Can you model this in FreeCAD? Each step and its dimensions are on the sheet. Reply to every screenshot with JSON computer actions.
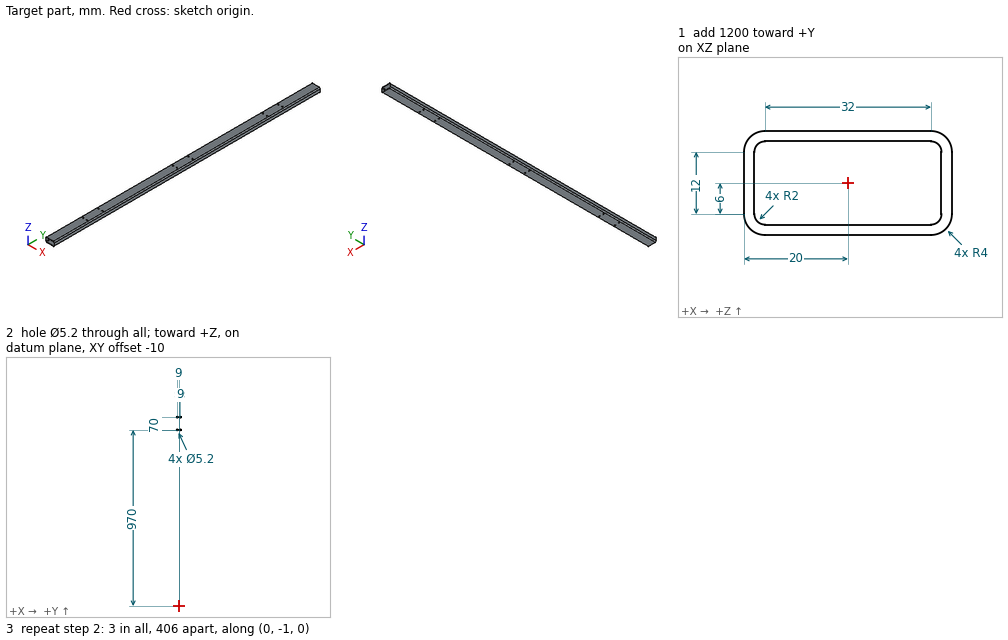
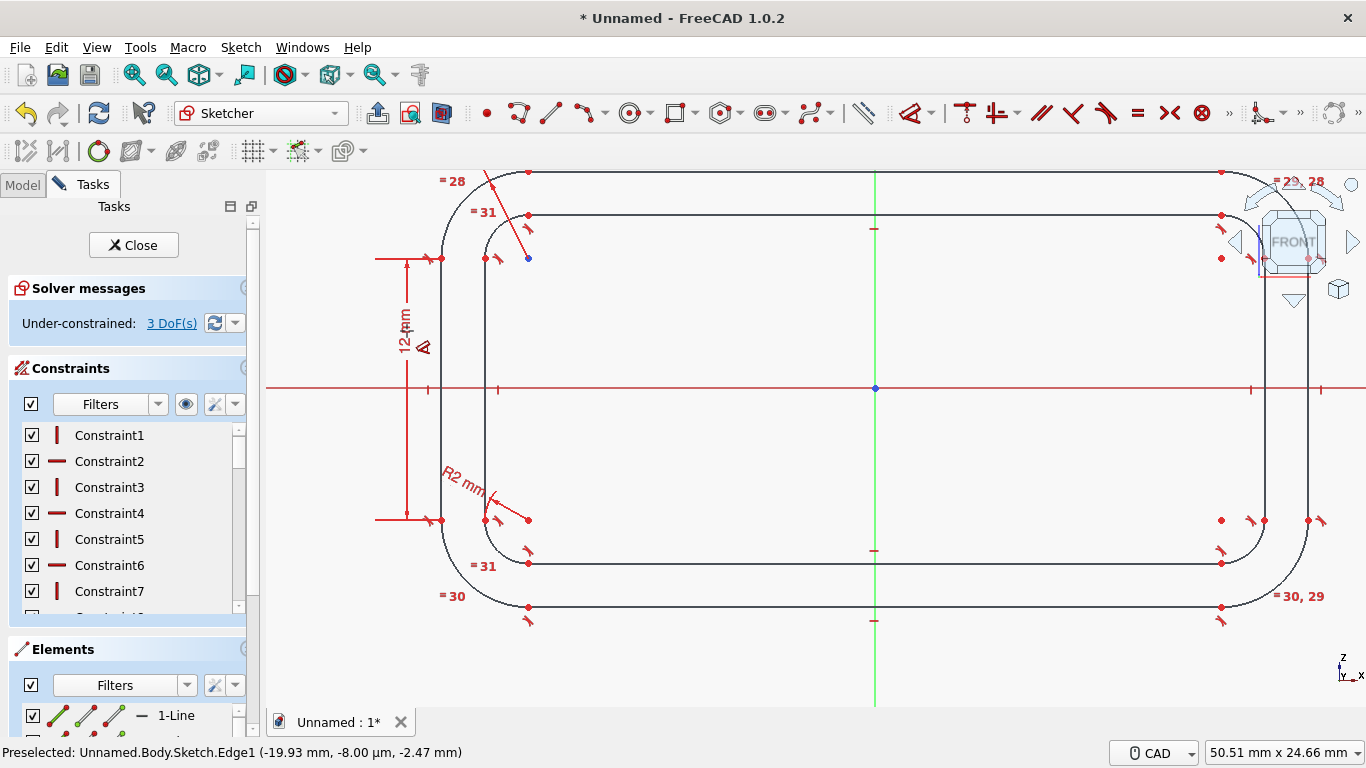
{"action": "scroll", "coordinate": [487, 541], "scroll_direction": "down", "scroll_amount": 2}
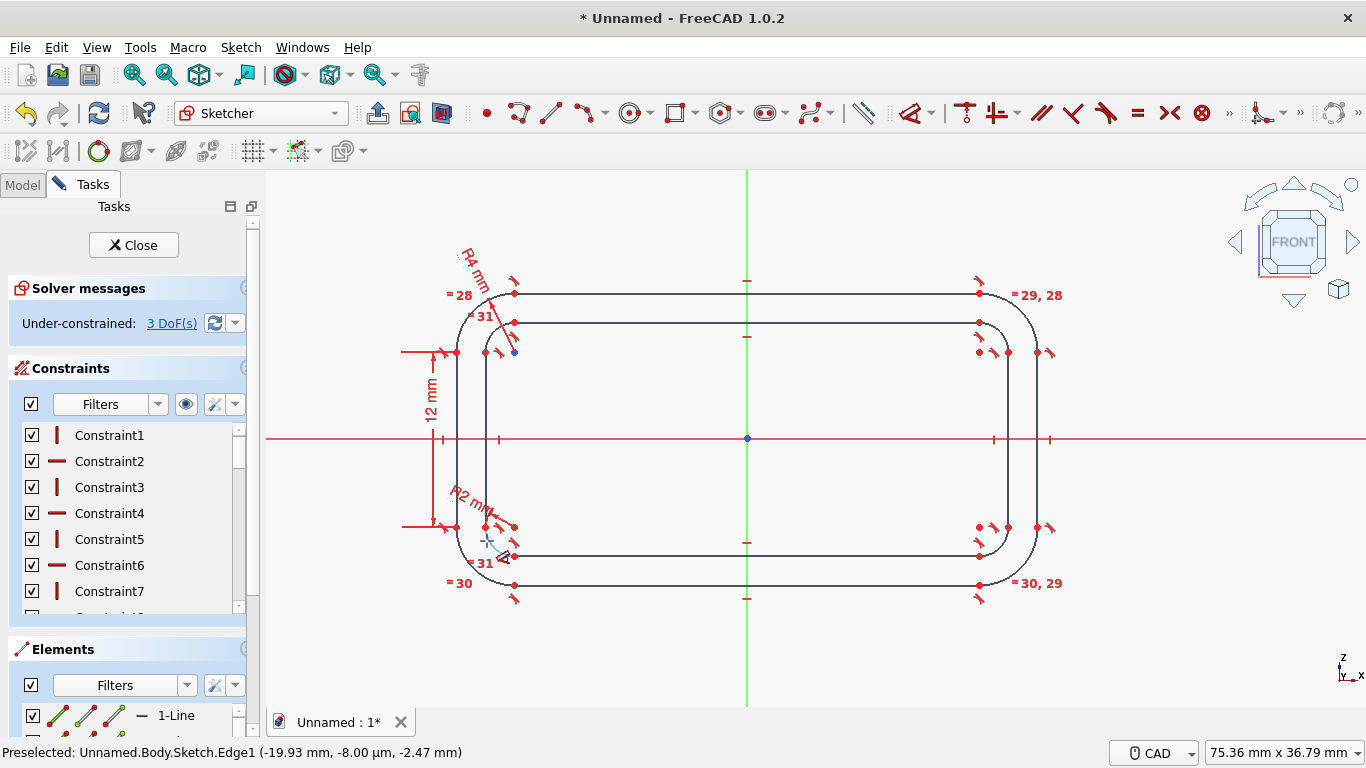
{"action": "left_click", "coordinate": [654, 294]}
{"action": "left_click", "coordinate": [640, 260]}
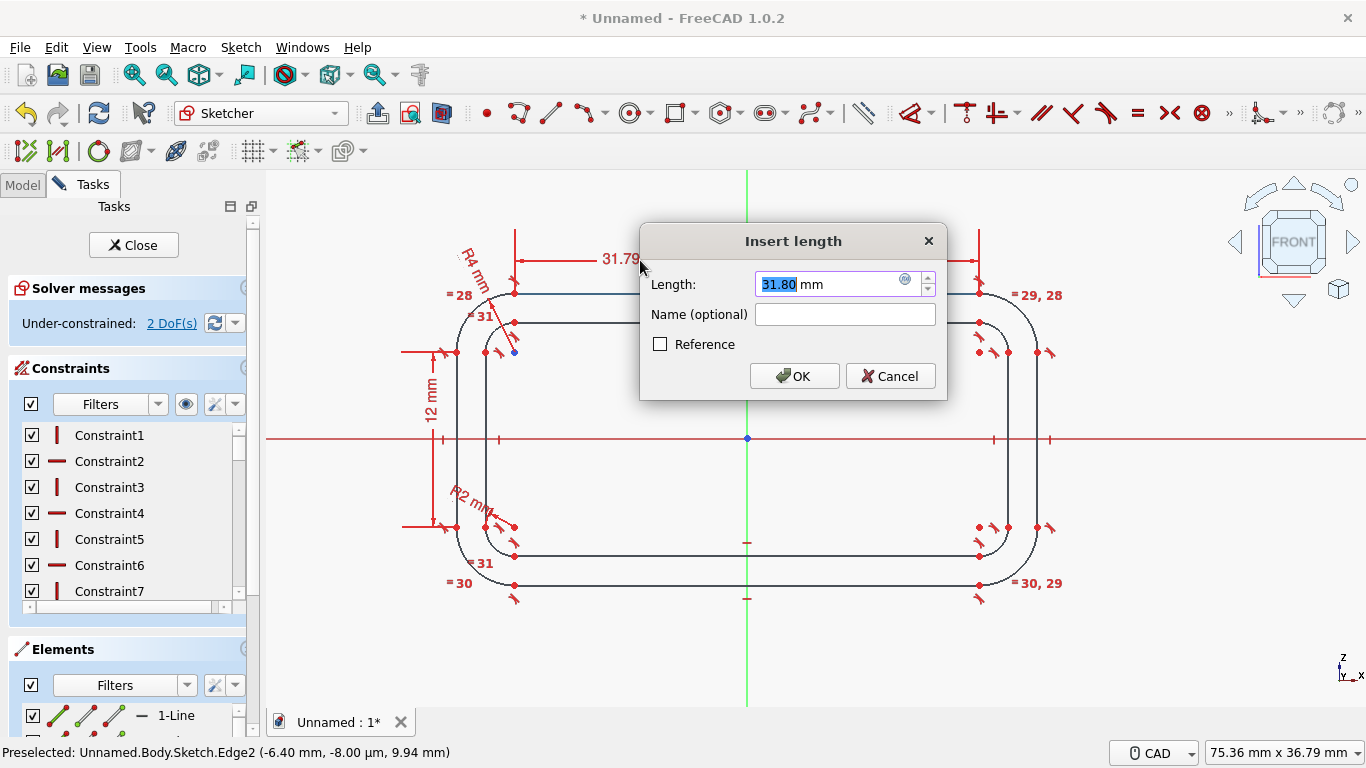
{"action": "type", "text": "32"}
{"action": "key", "text": "Return"}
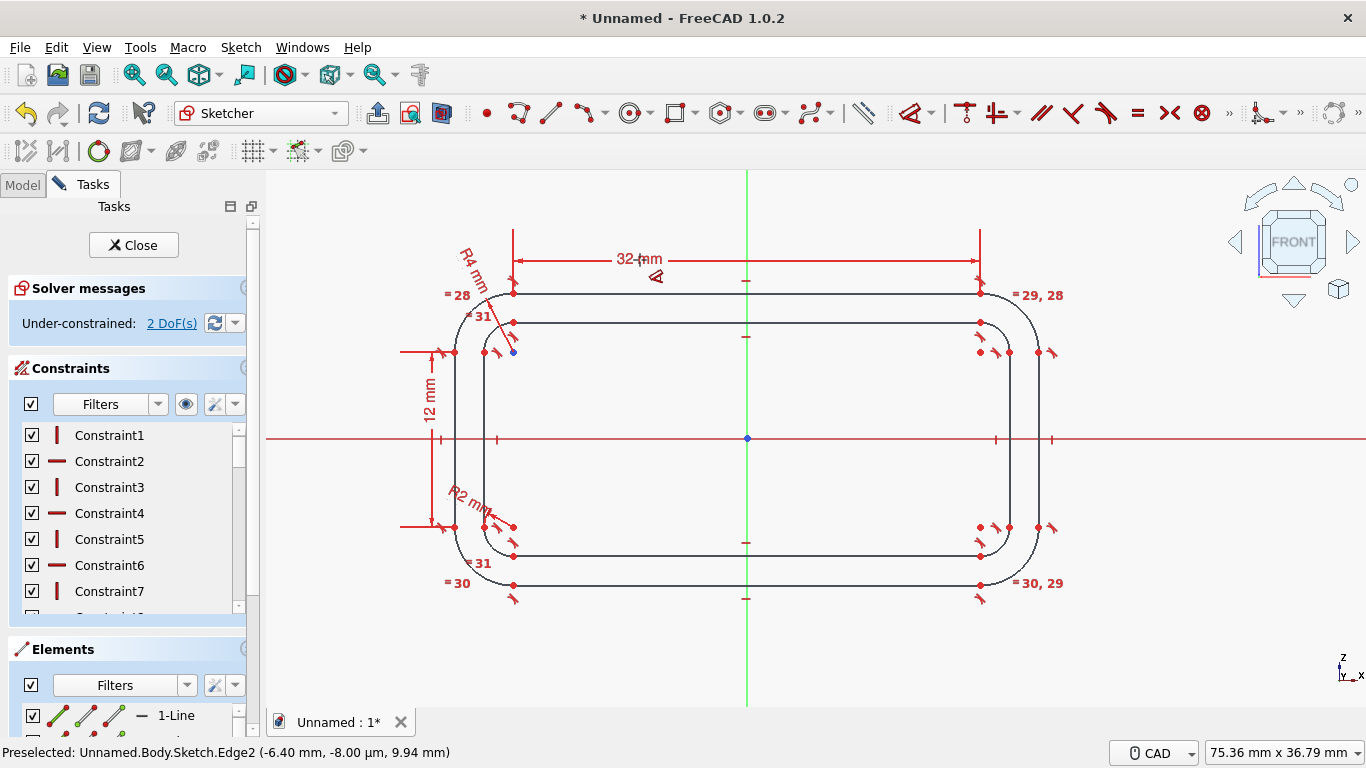
{"action": "left_click", "coordinate": [455, 527]}
{"action": "left_click", "coordinate": [421, 463]}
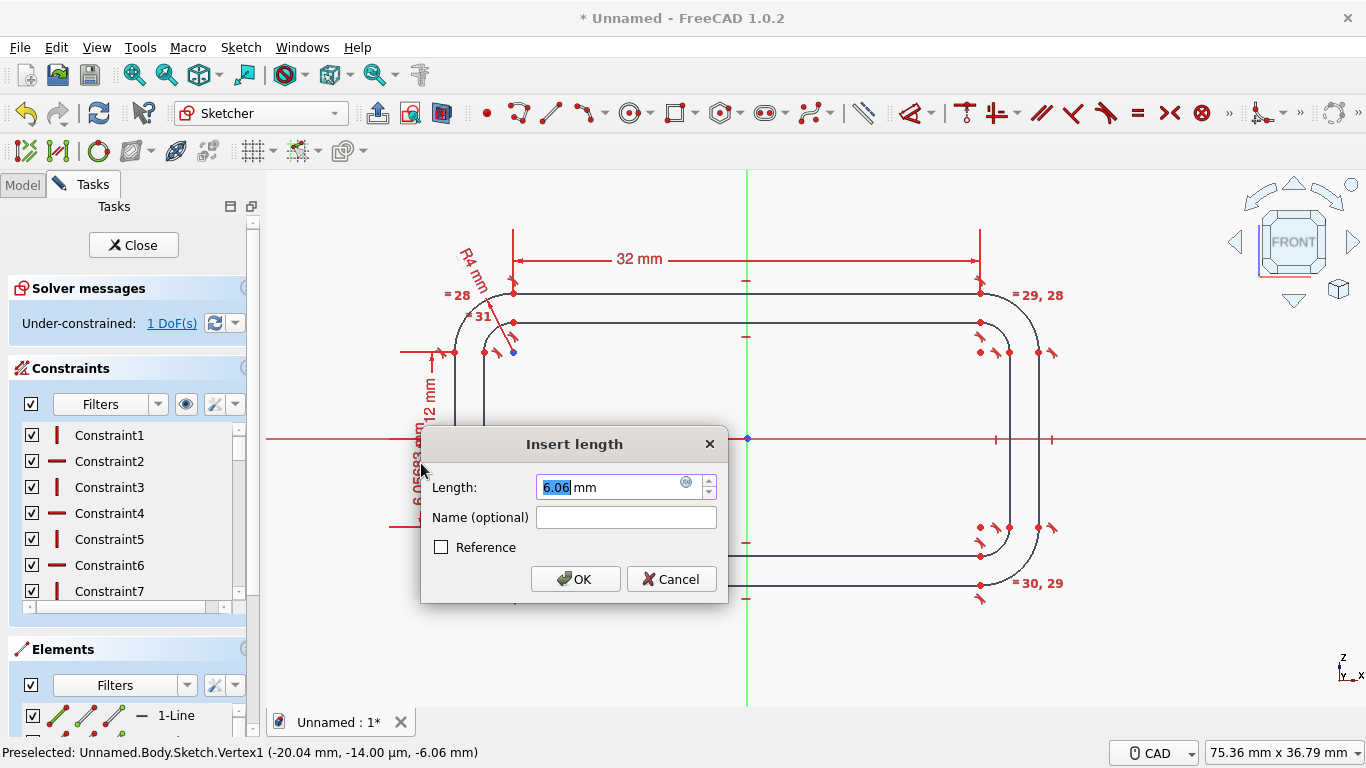
{"action": "type", "text": "6"}
{"action": "key", "text": "Return"}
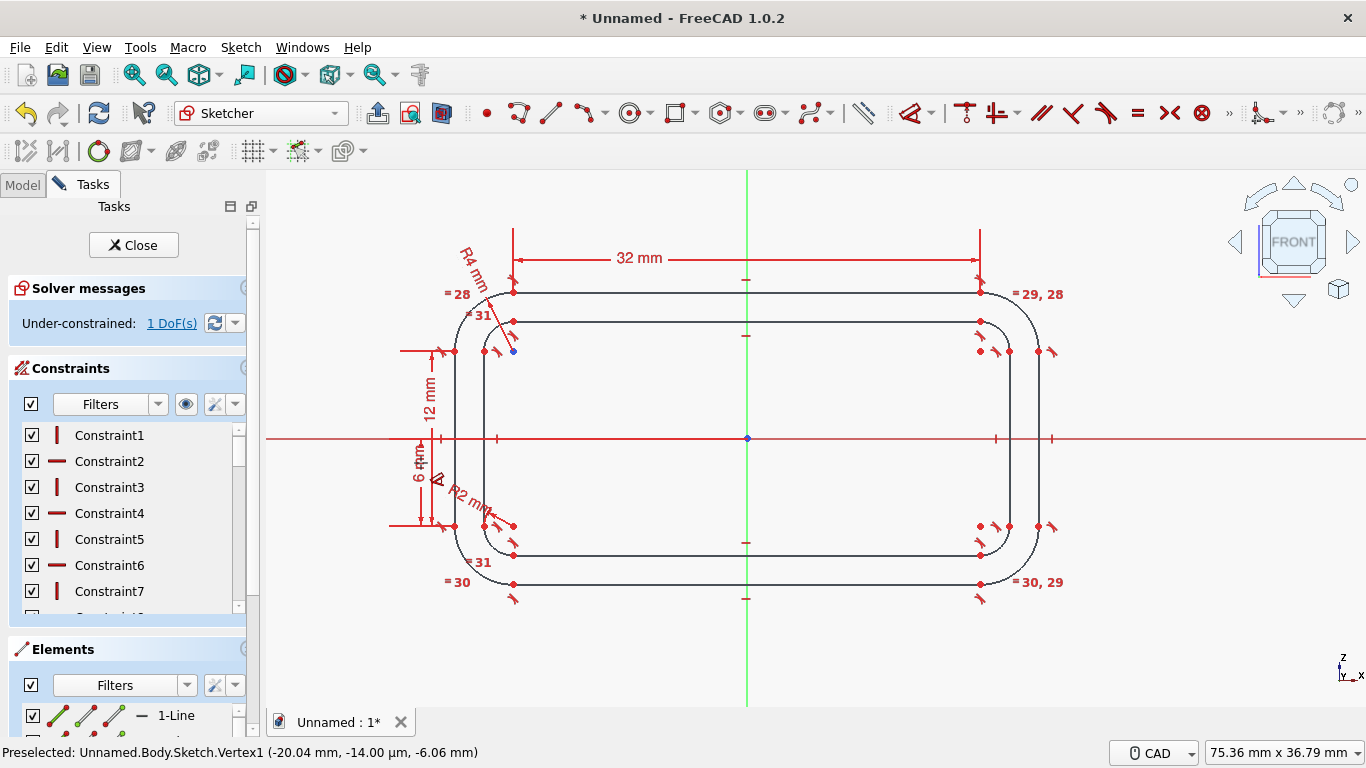
{"action": "left_click", "coordinate": [455, 526]}
{"action": "left_click", "coordinate": [601, 405]}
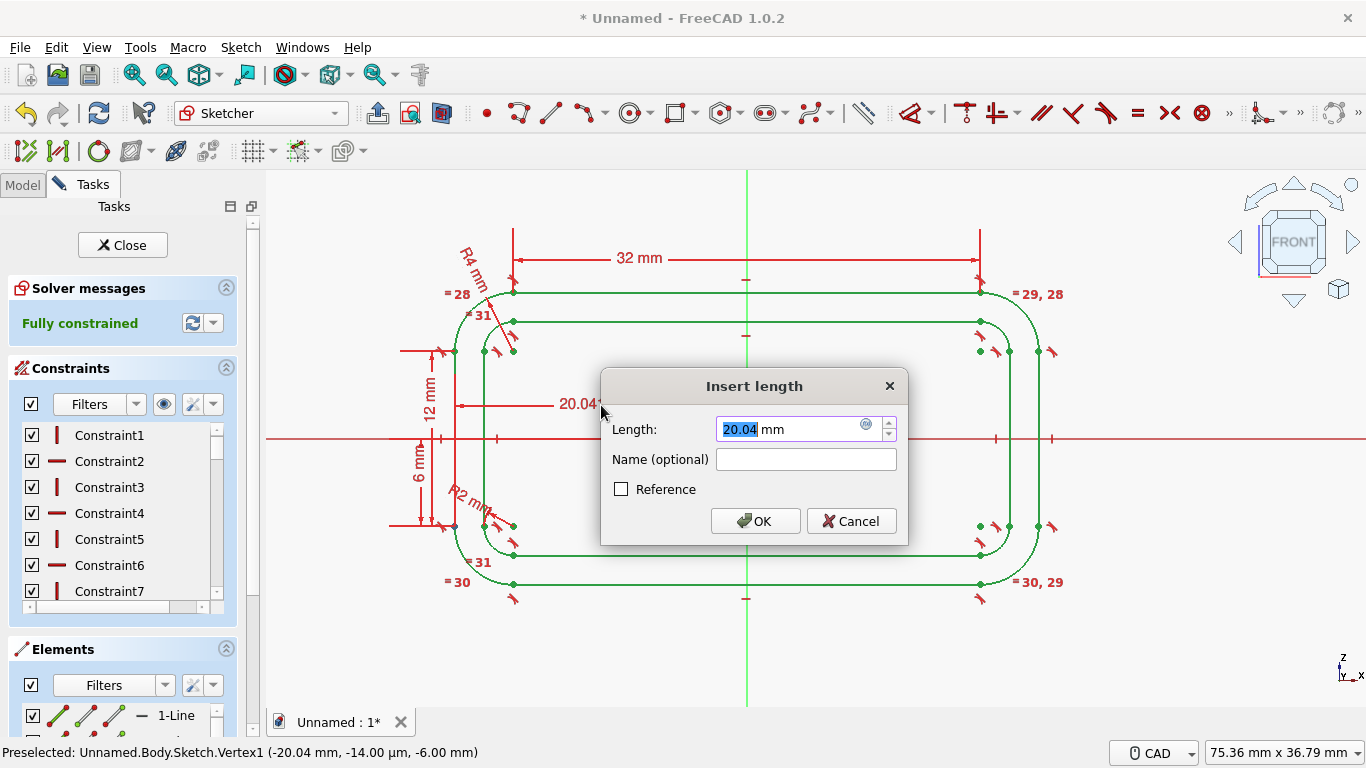
{"action": "type", "text": "20"}
{"action": "key", "text": "Return"}
{"action": "key", "text": "Escape"}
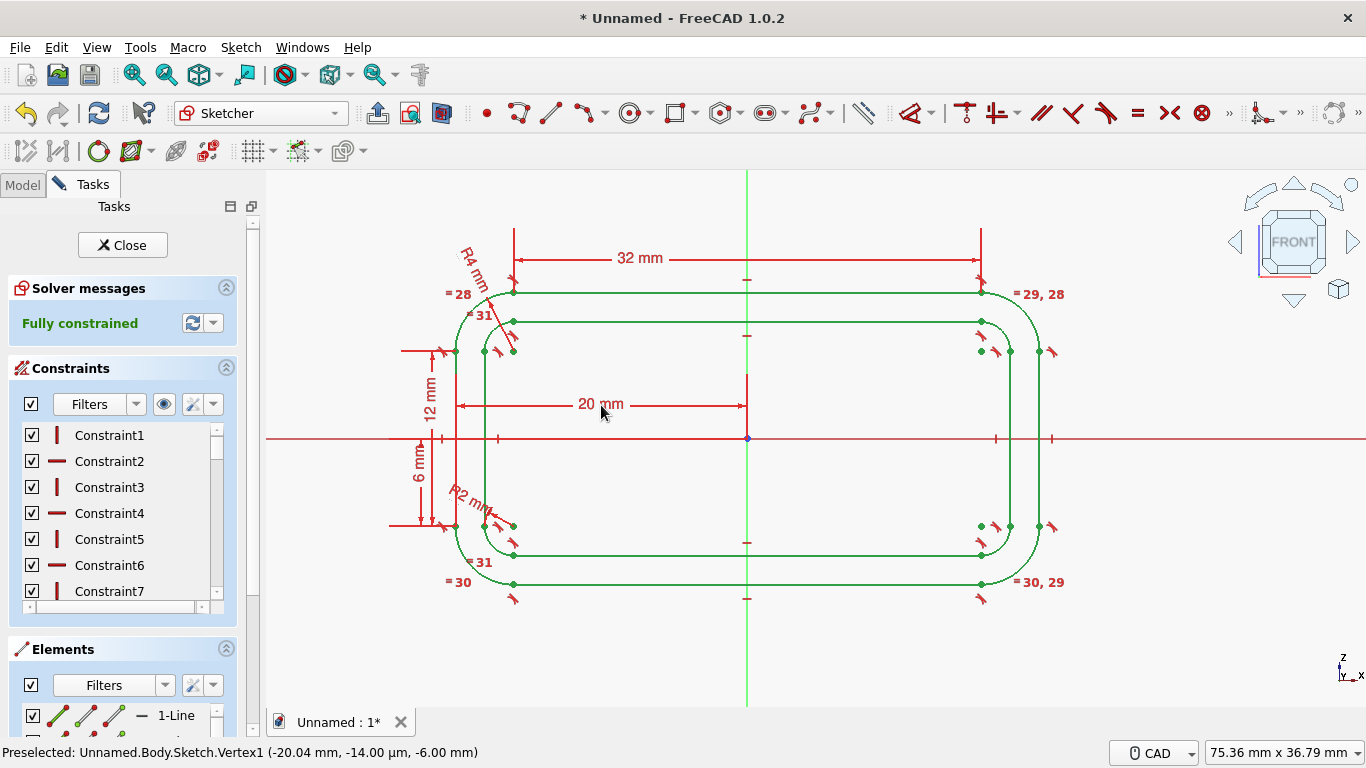
{"action": "left_click", "coordinate": [123, 245]}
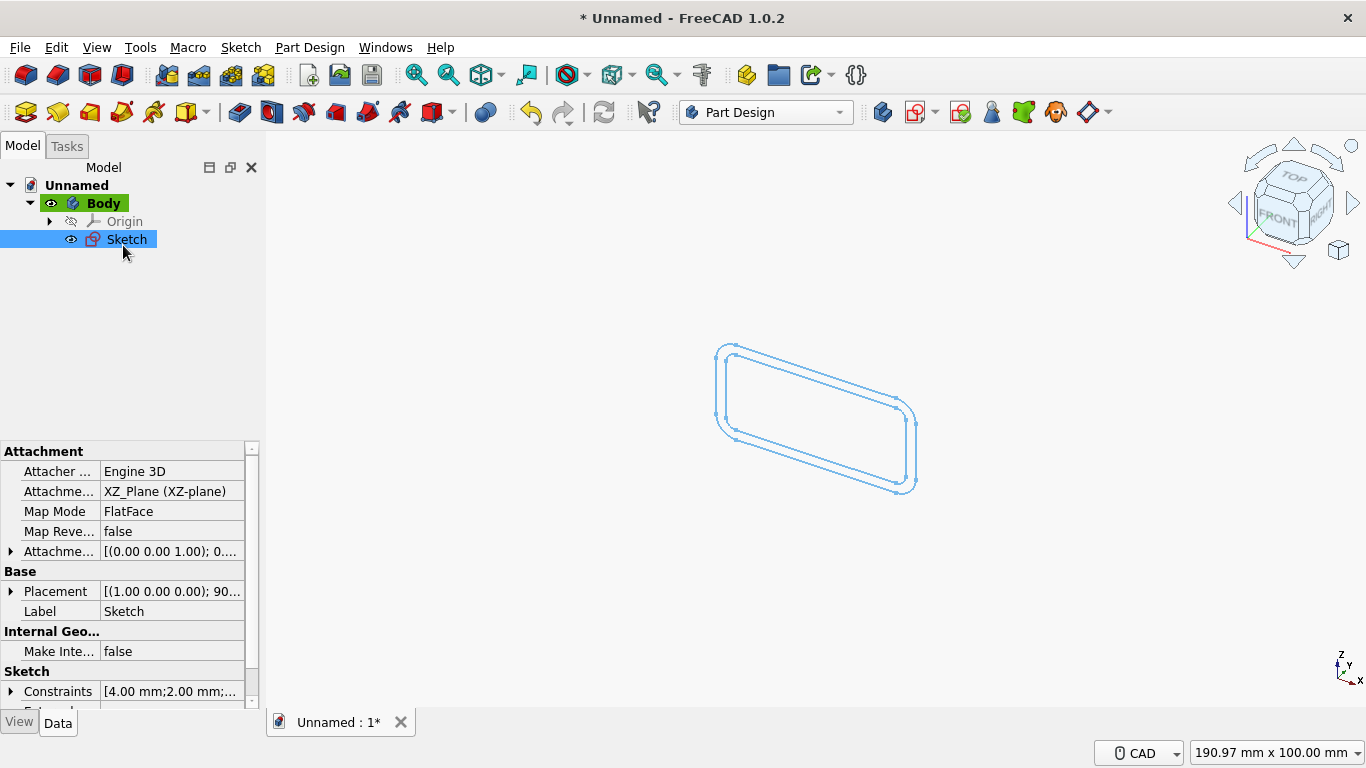
{"action": "left_click", "coordinate": [26, 112]}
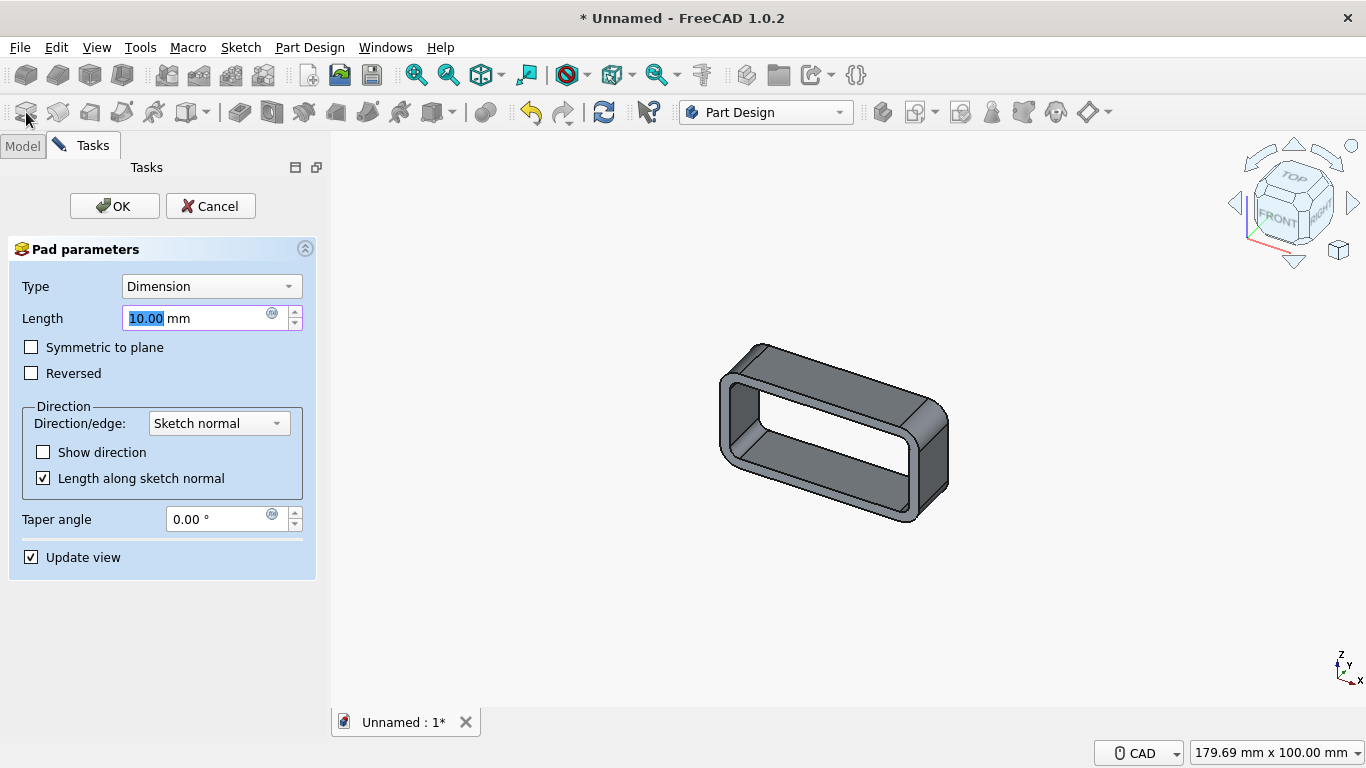
{"action": "type", "text": "1200"}
{"action": "key", "text": "Tab"}